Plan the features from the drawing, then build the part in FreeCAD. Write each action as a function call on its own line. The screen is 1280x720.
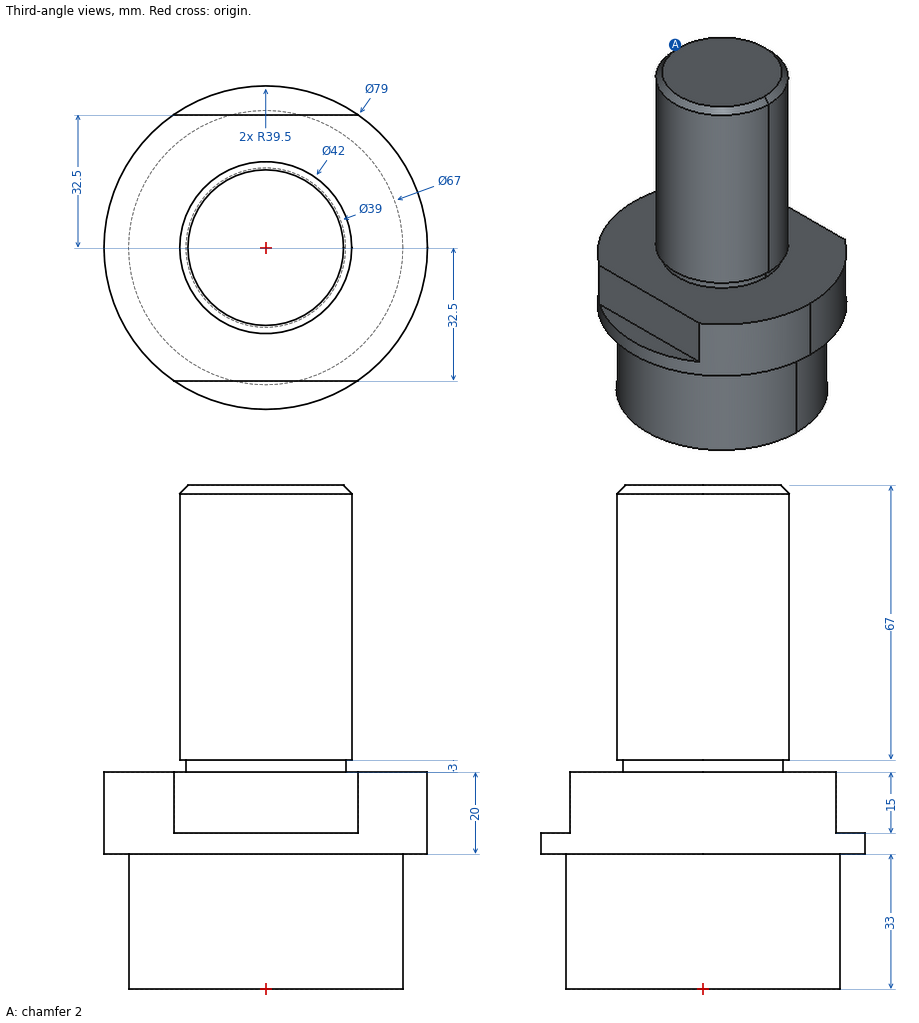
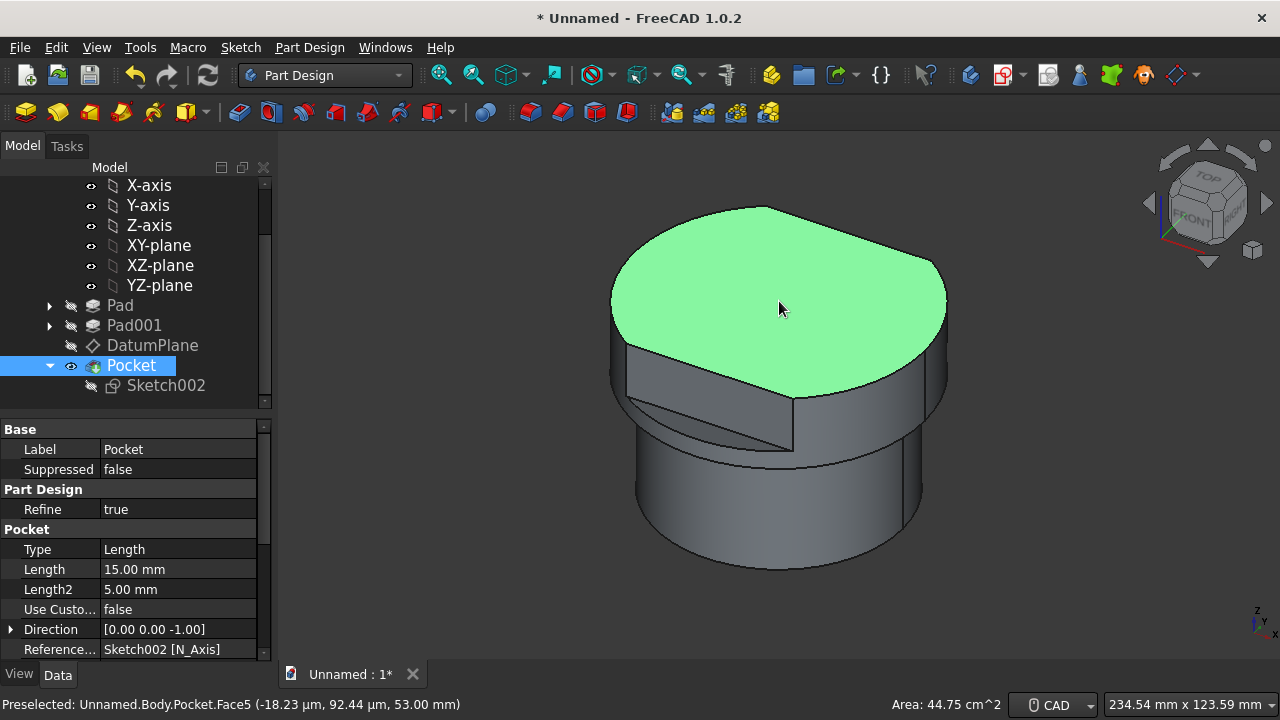
click(1004, 76)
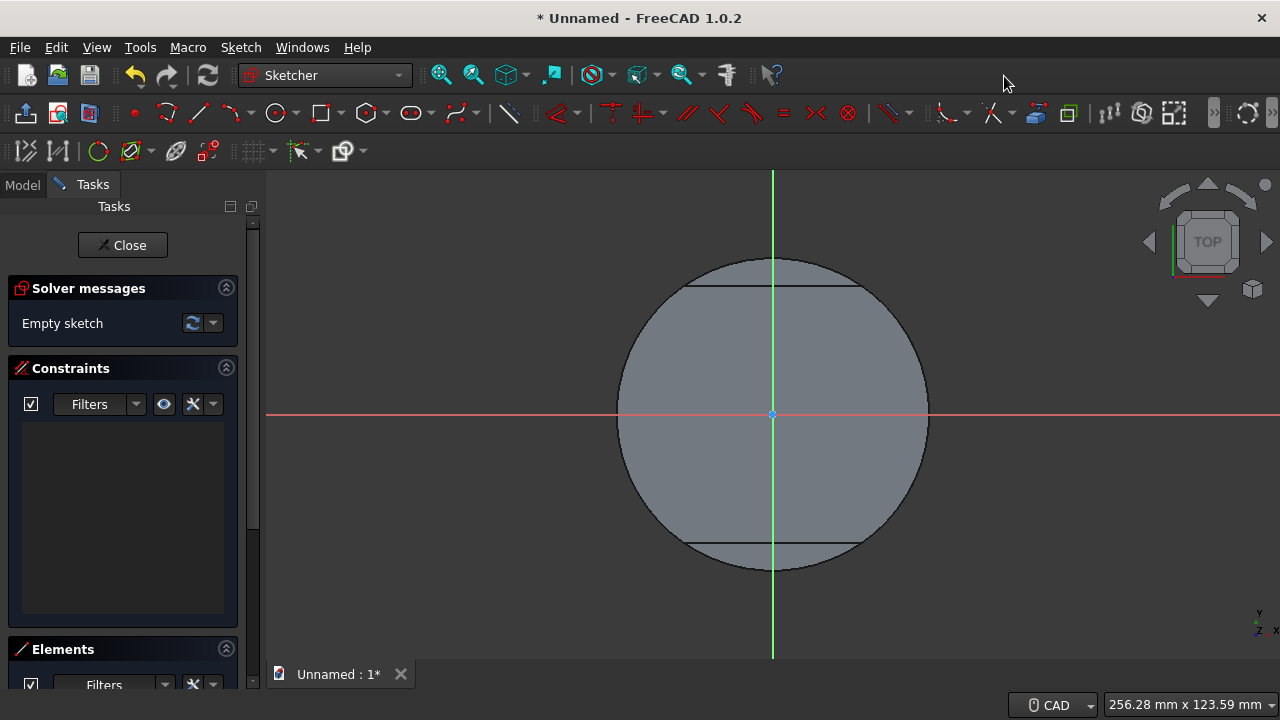
scroll(856, 415, up, 3)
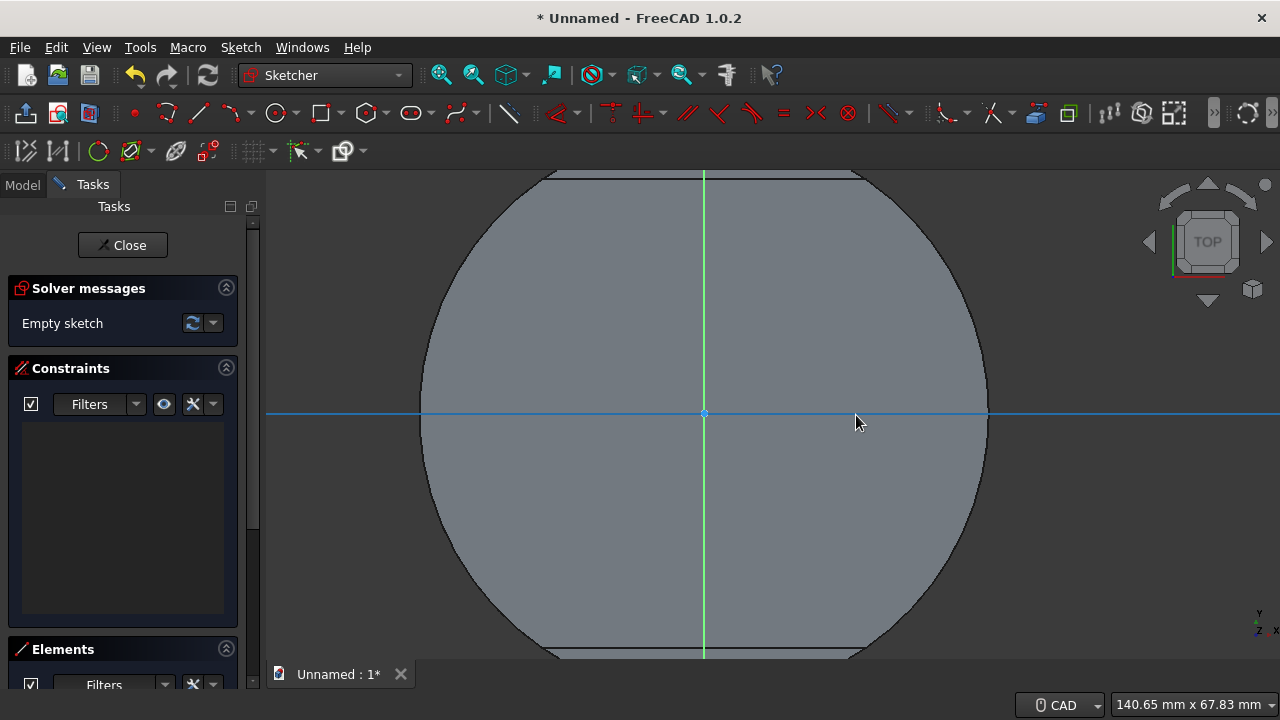
click(276, 114)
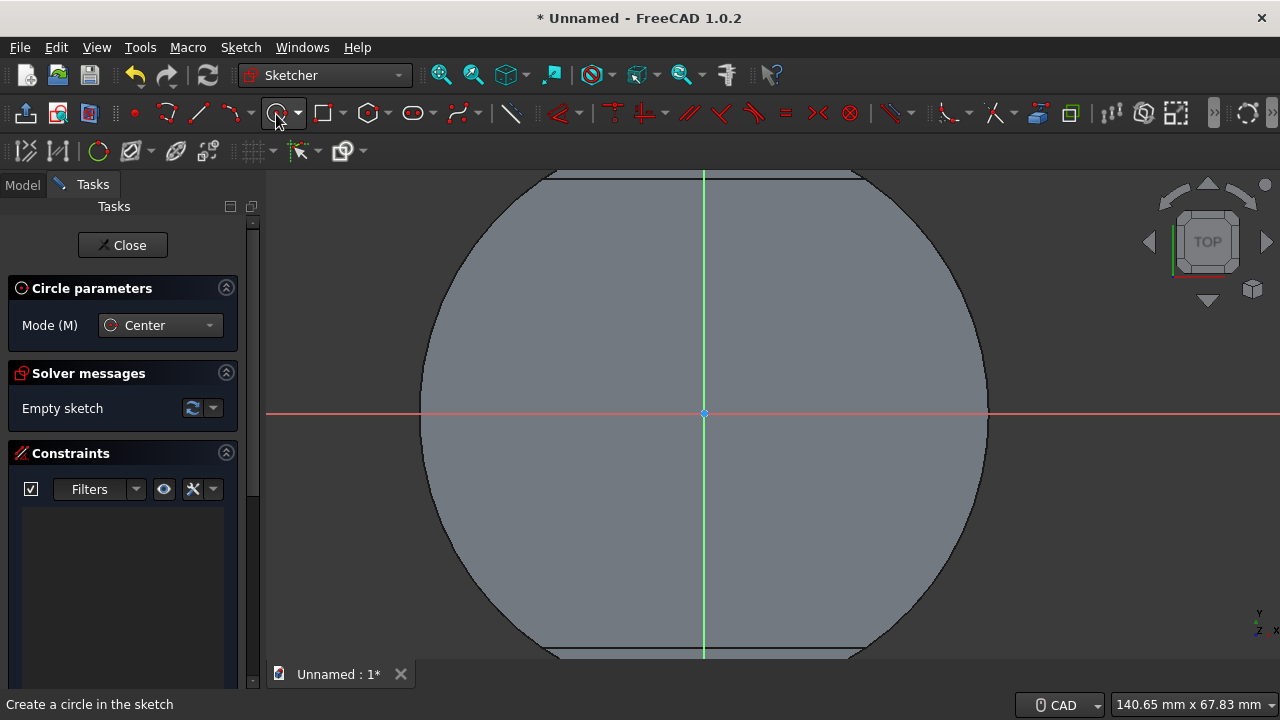
click(704, 414)
move(803, 314)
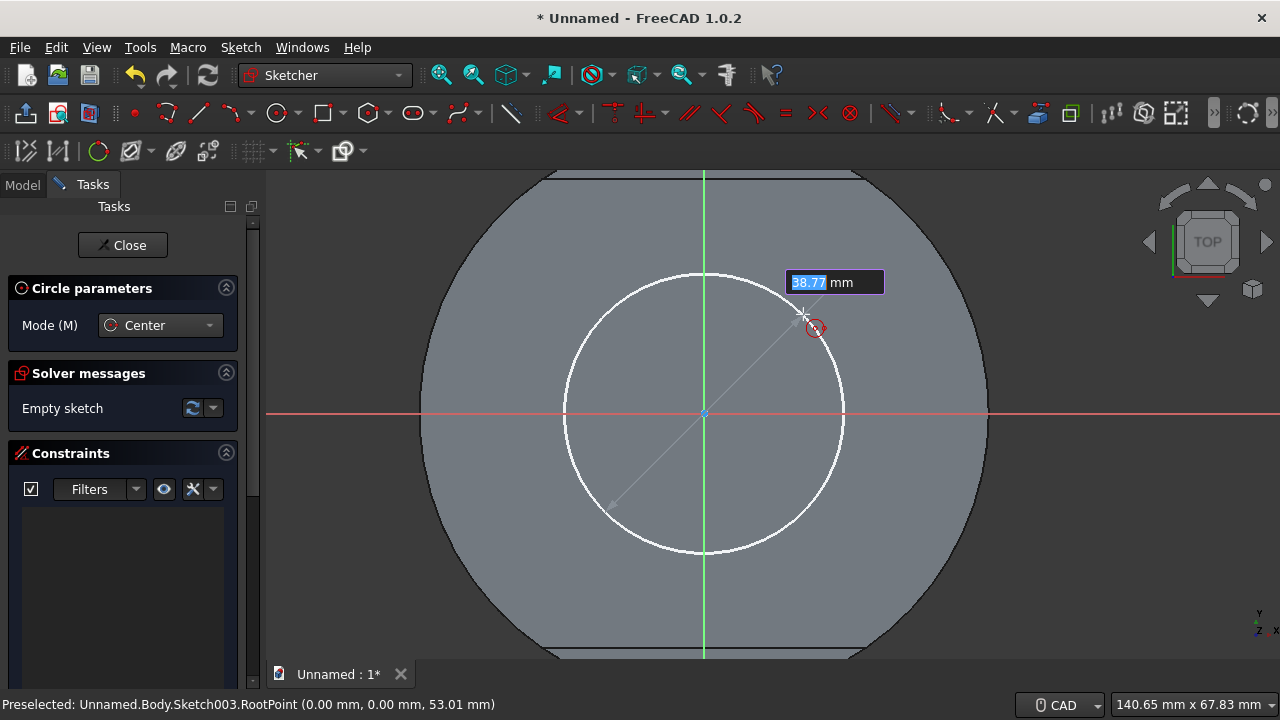
text(39)
key(Return)
key(Escape)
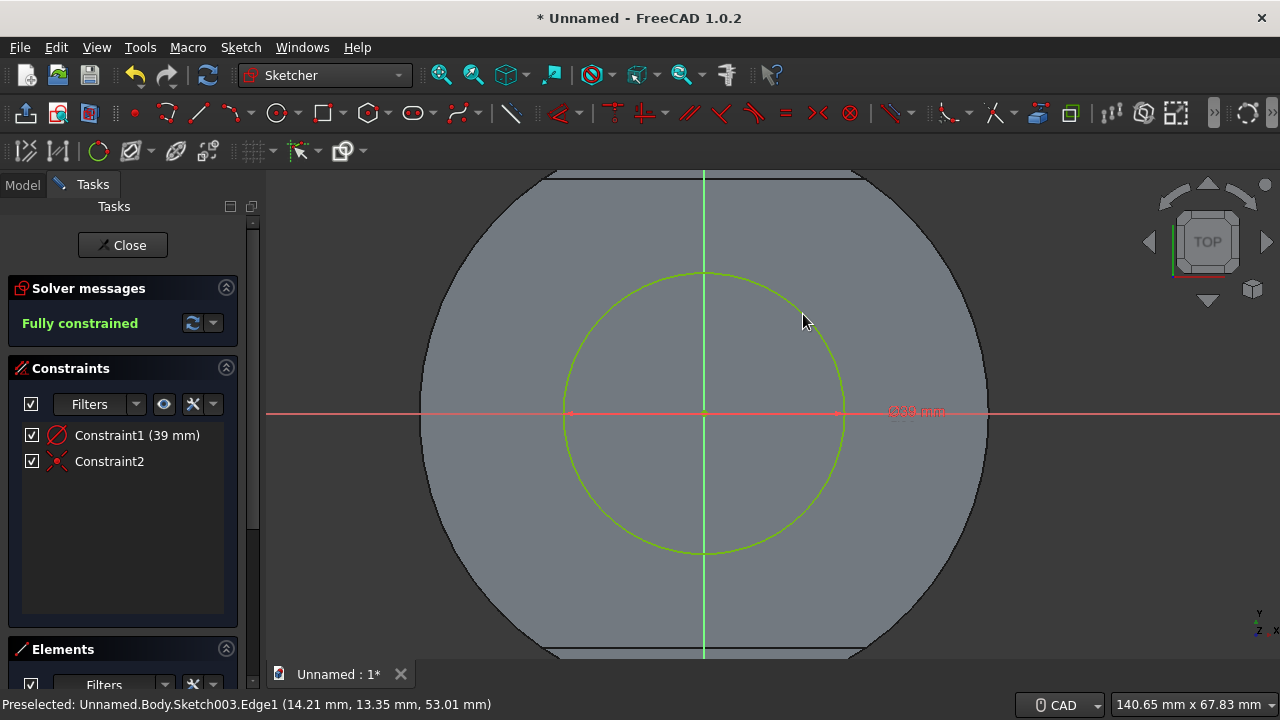
click(123, 245)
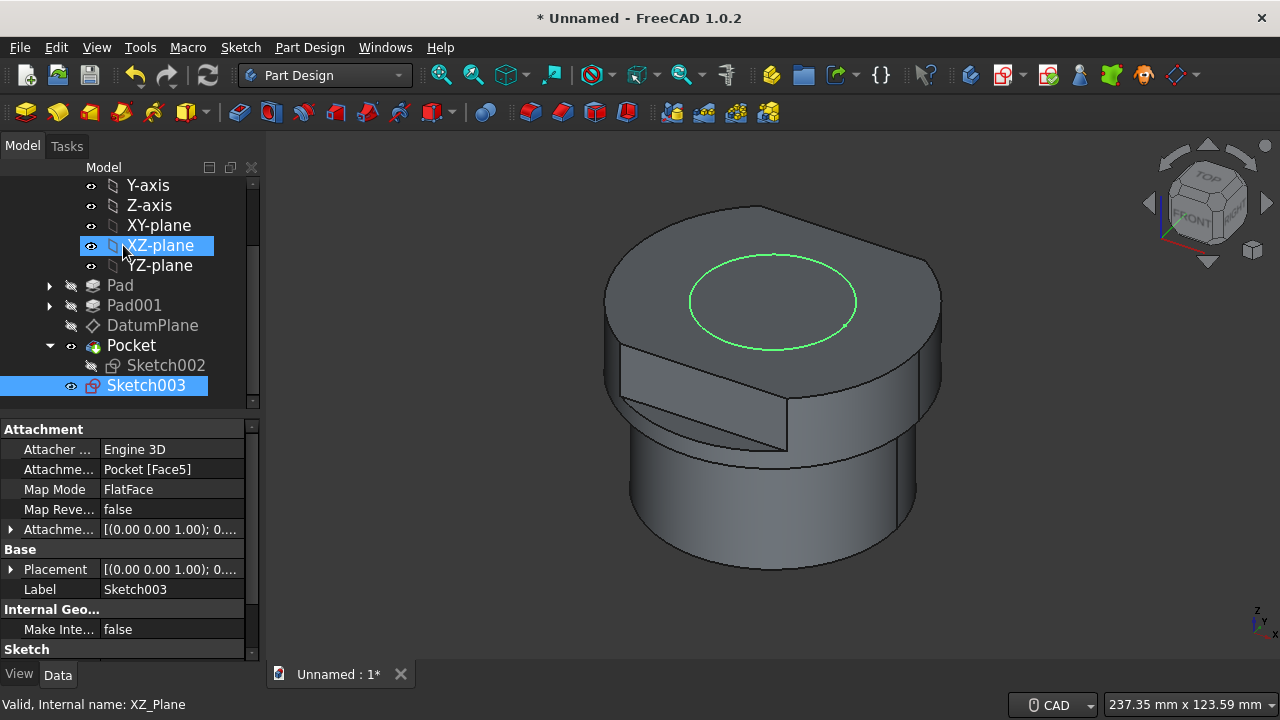
click(26, 112)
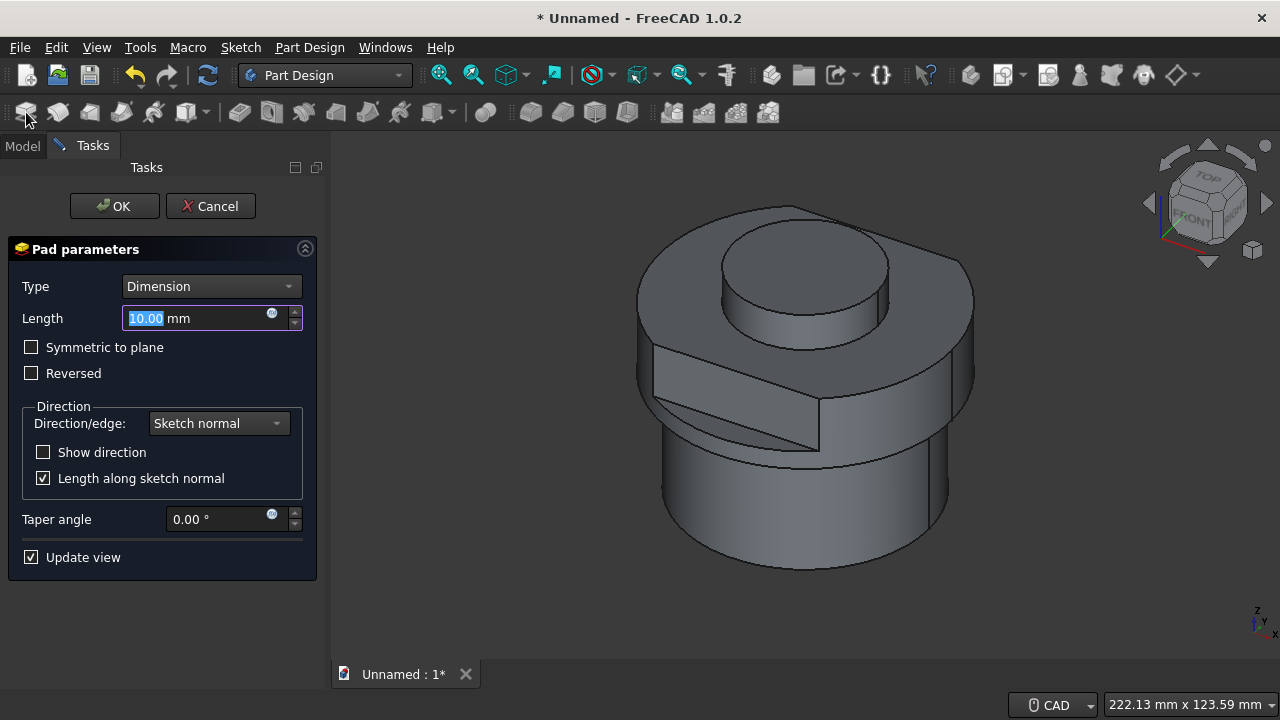
text(3)
key(Tab)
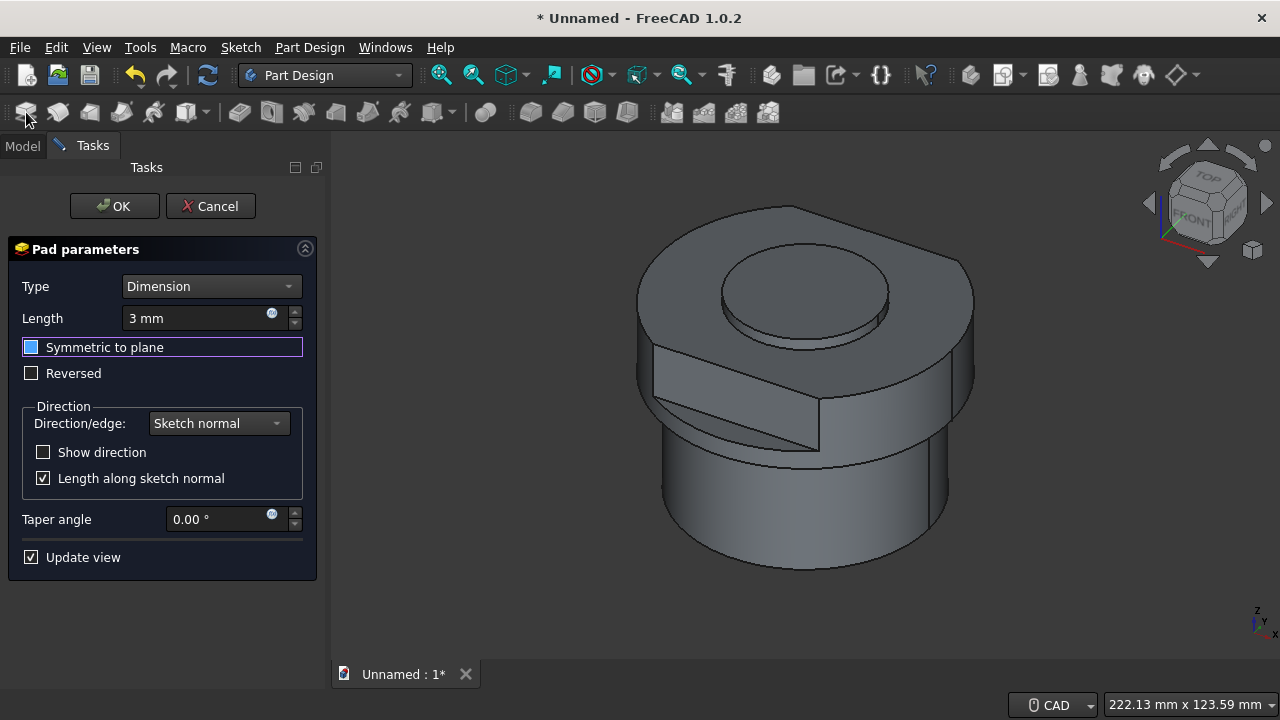
click(115, 206)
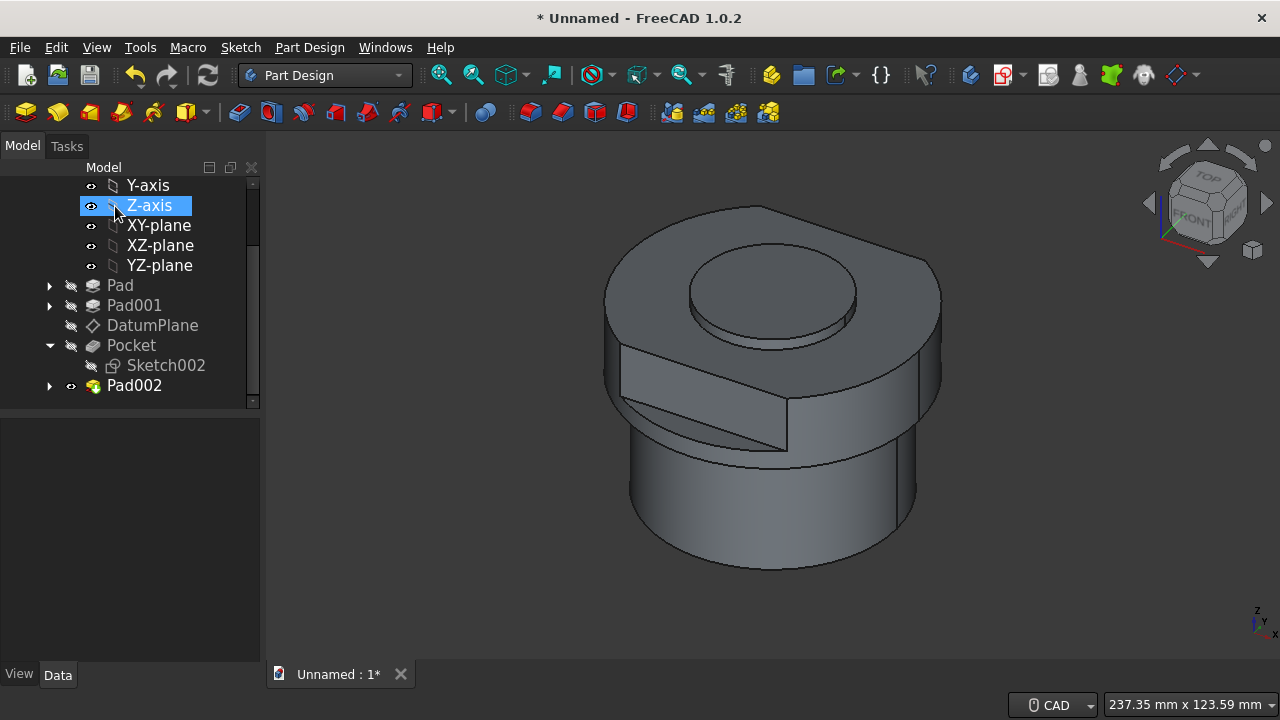
click(773, 291)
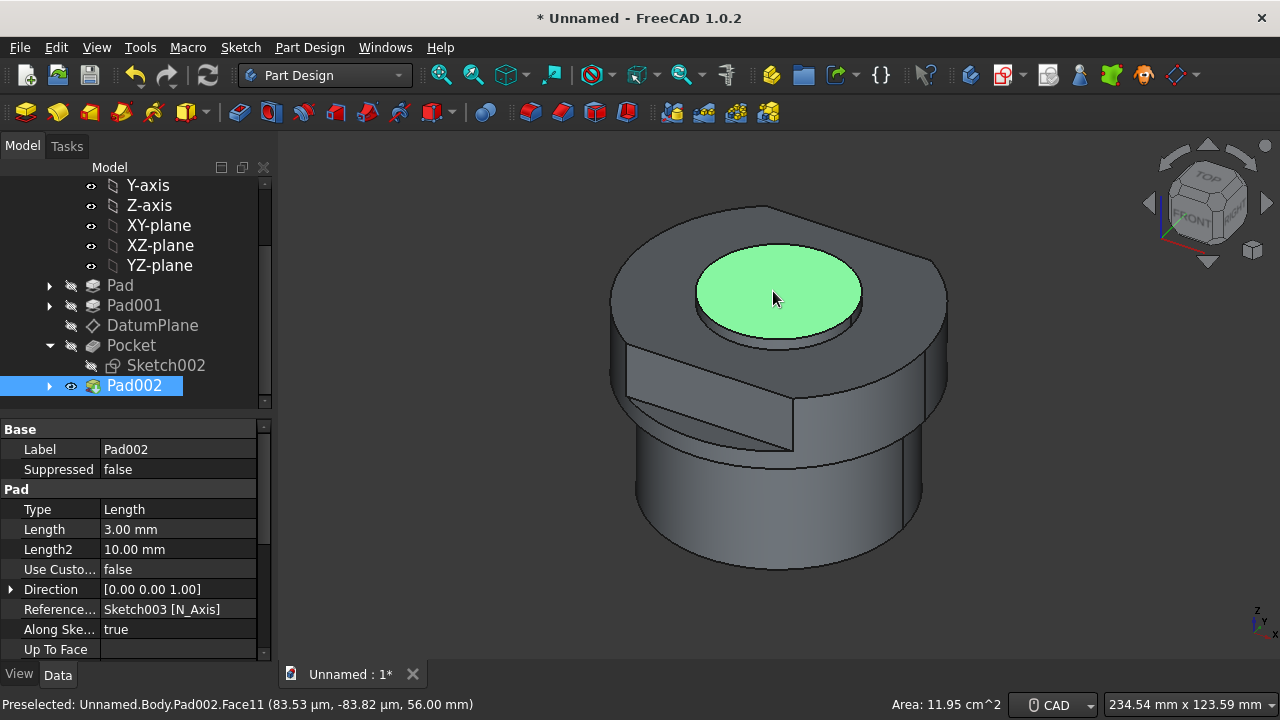
click(1004, 76)